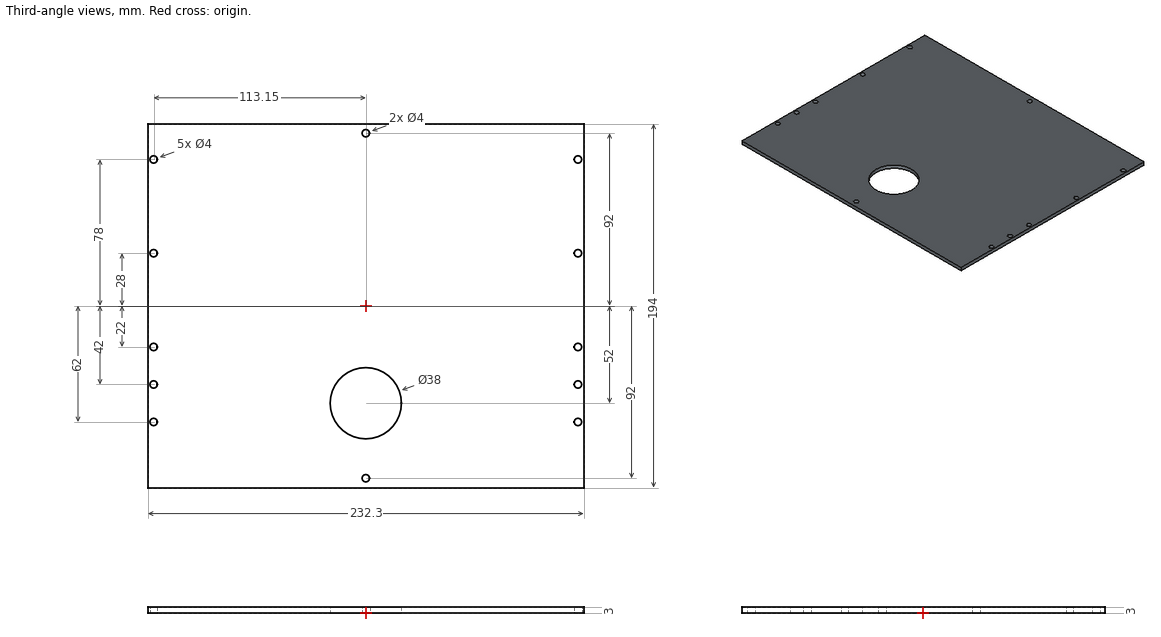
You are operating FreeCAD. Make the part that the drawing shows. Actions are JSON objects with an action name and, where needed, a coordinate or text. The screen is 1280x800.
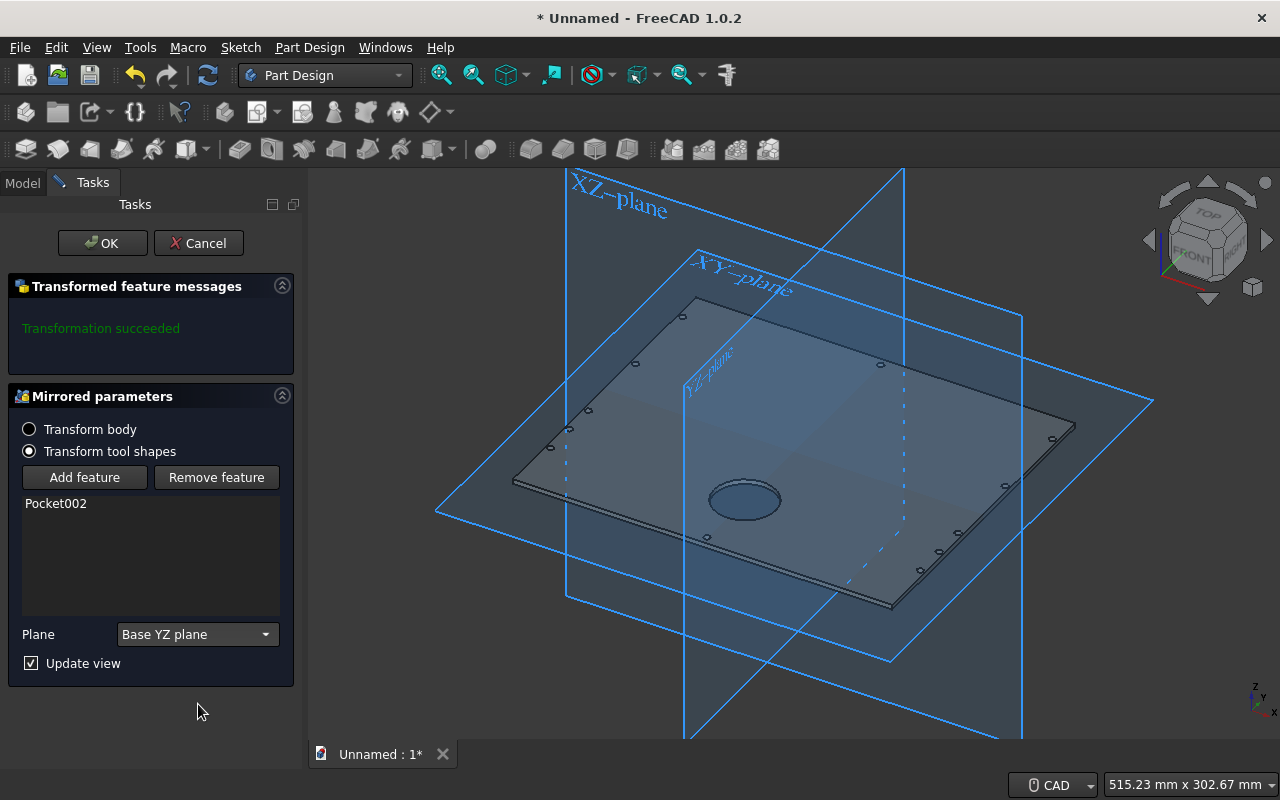
{"action": "left_click", "coordinate": [103, 243]}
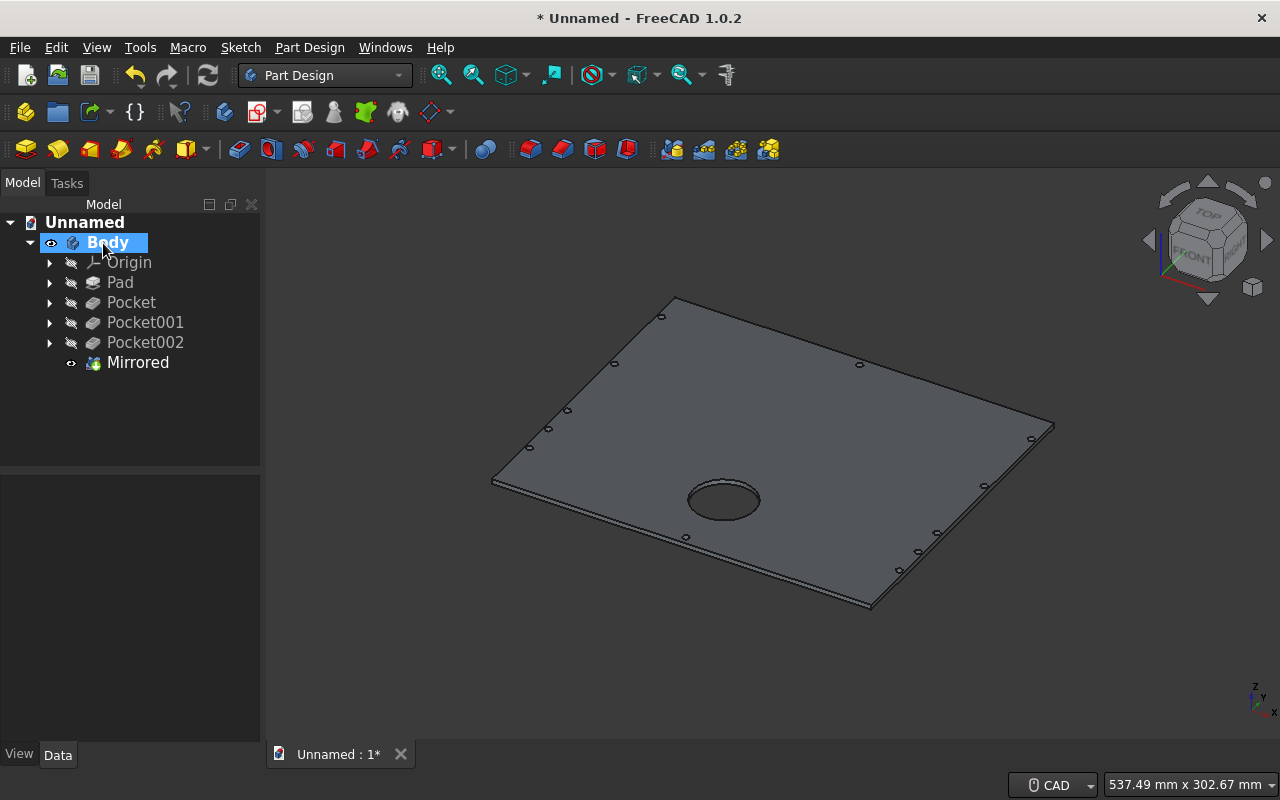
{"action": "key", "text": "0"}